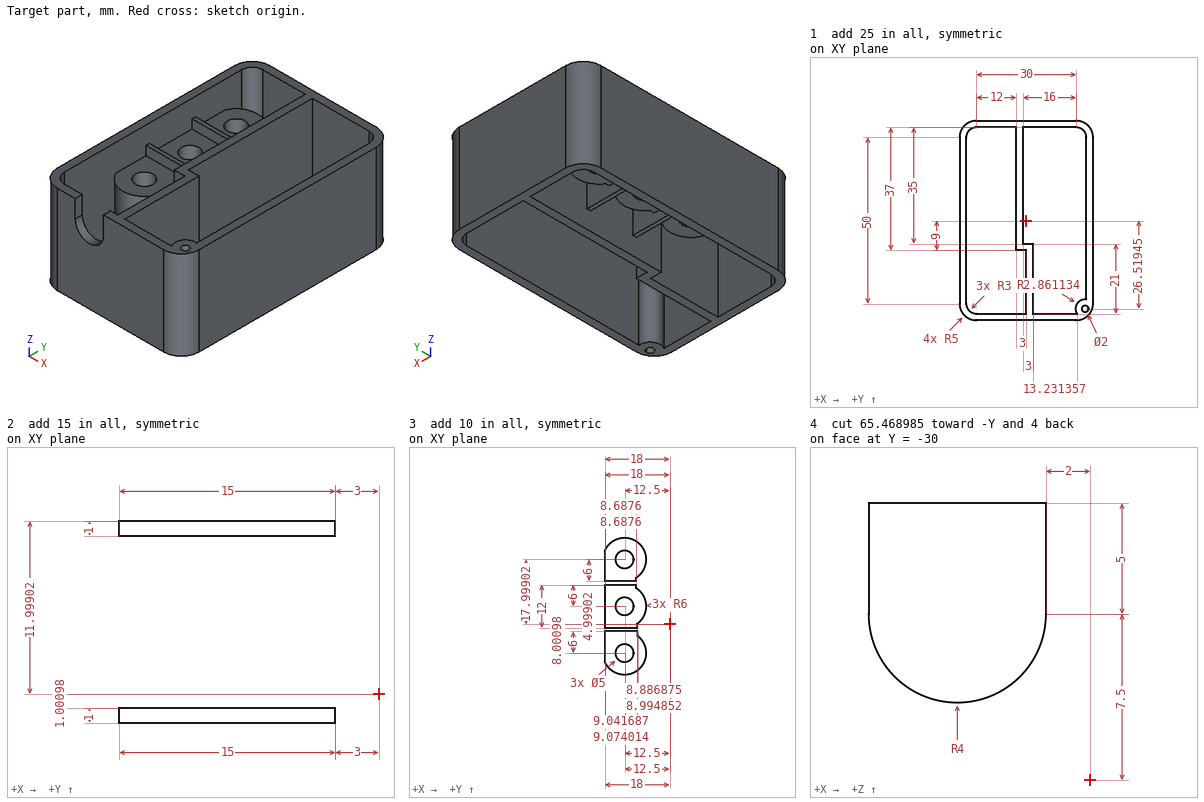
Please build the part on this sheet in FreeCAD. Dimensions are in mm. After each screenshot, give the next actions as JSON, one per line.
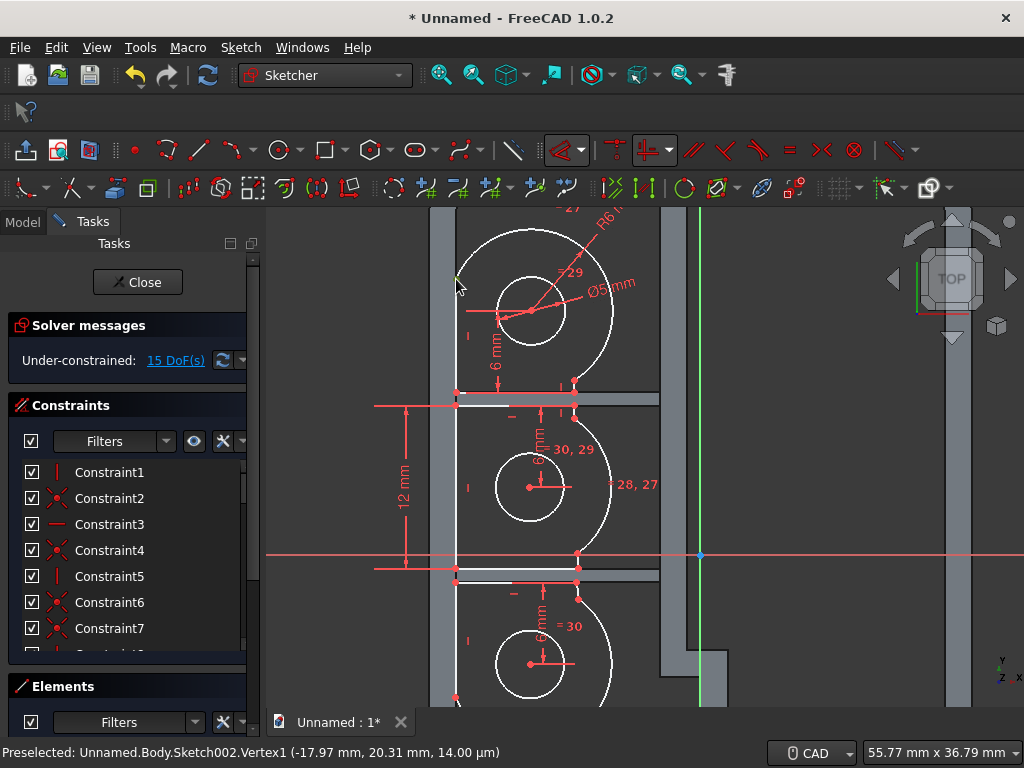
{"action": "key", "text": "l"}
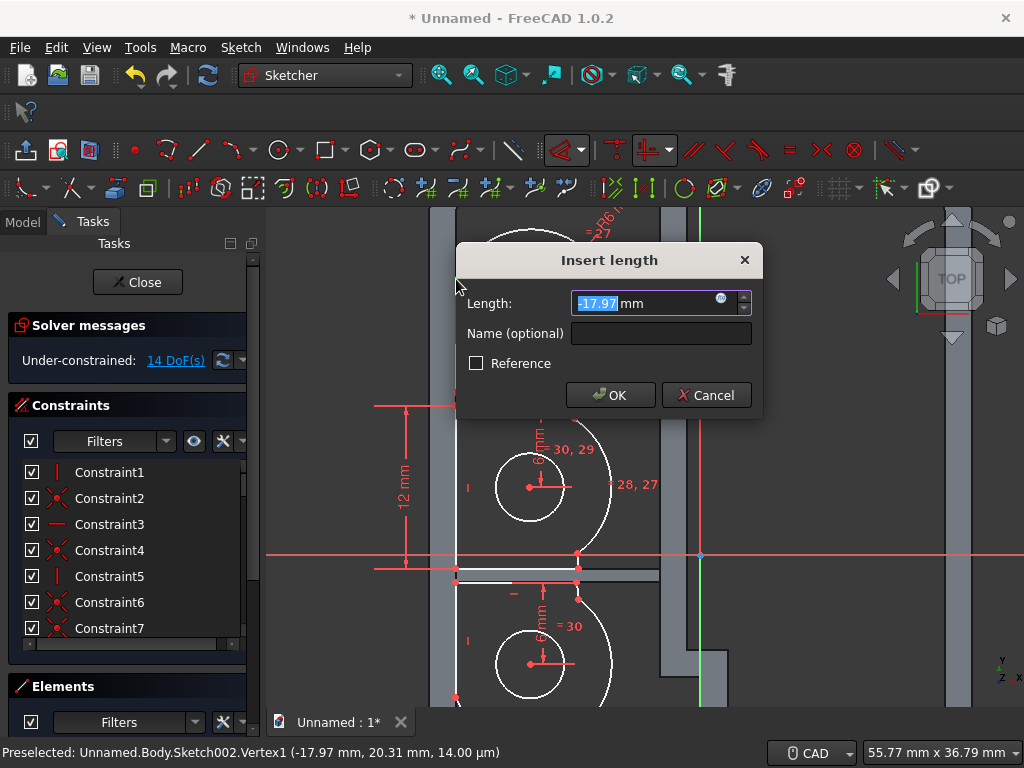
{"action": "type", "text": "-18"}
{"action": "key", "text": "Return"}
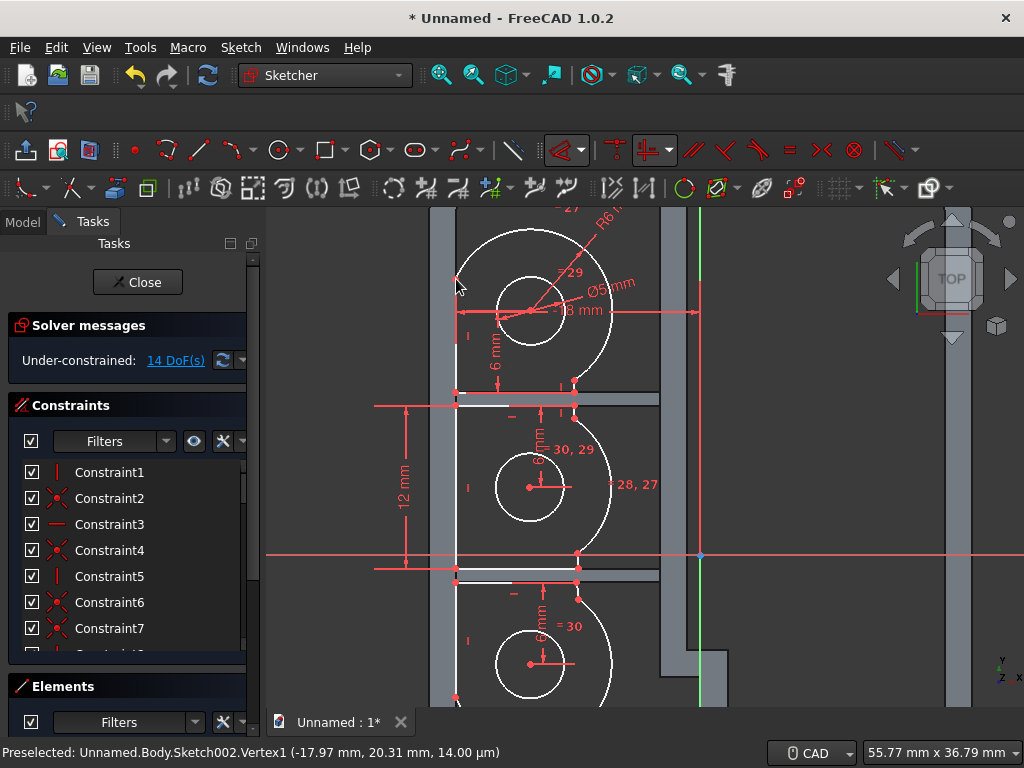
{"action": "left_click", "coordinate": [456, 406]}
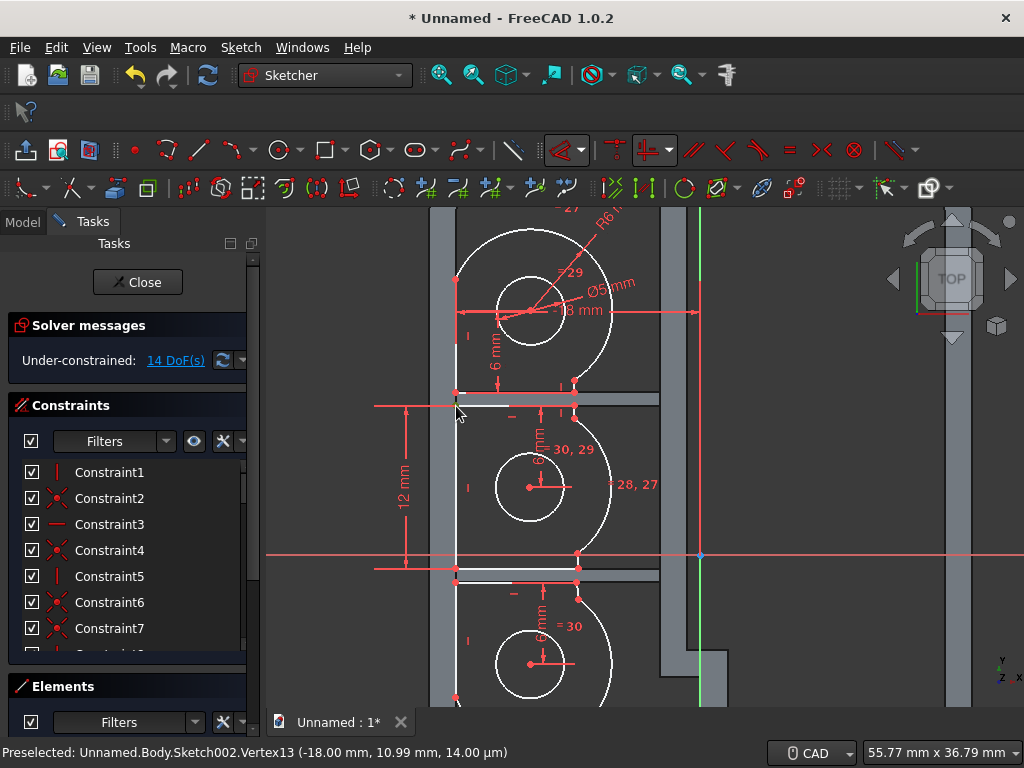
{"action": "left_click", "coordinate": [584, 150]}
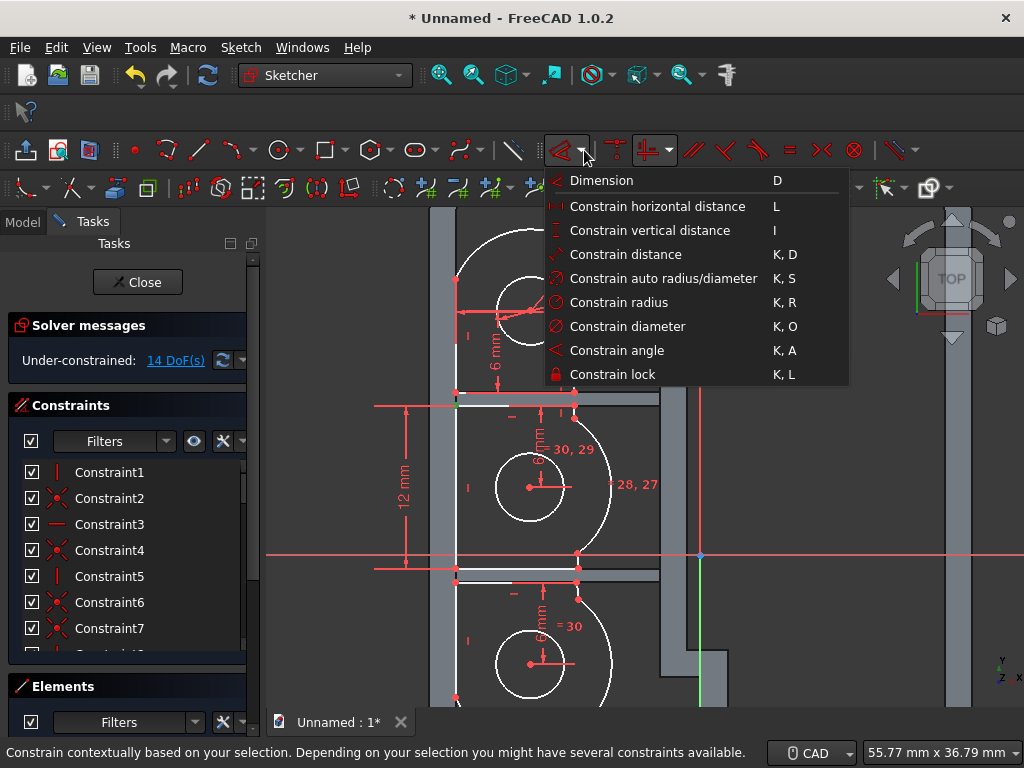
{"action": "left_click", "coordinate": [697, 206]}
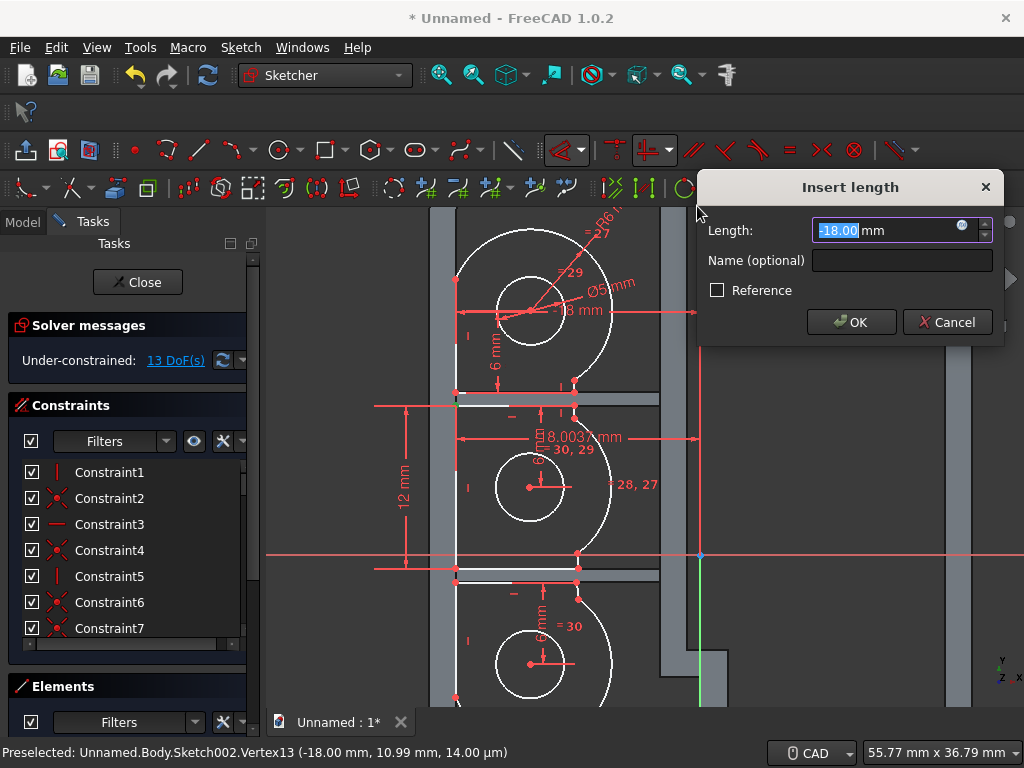
{"action": "type", "text": "-18"}
{"action": "key", "text": "Return"}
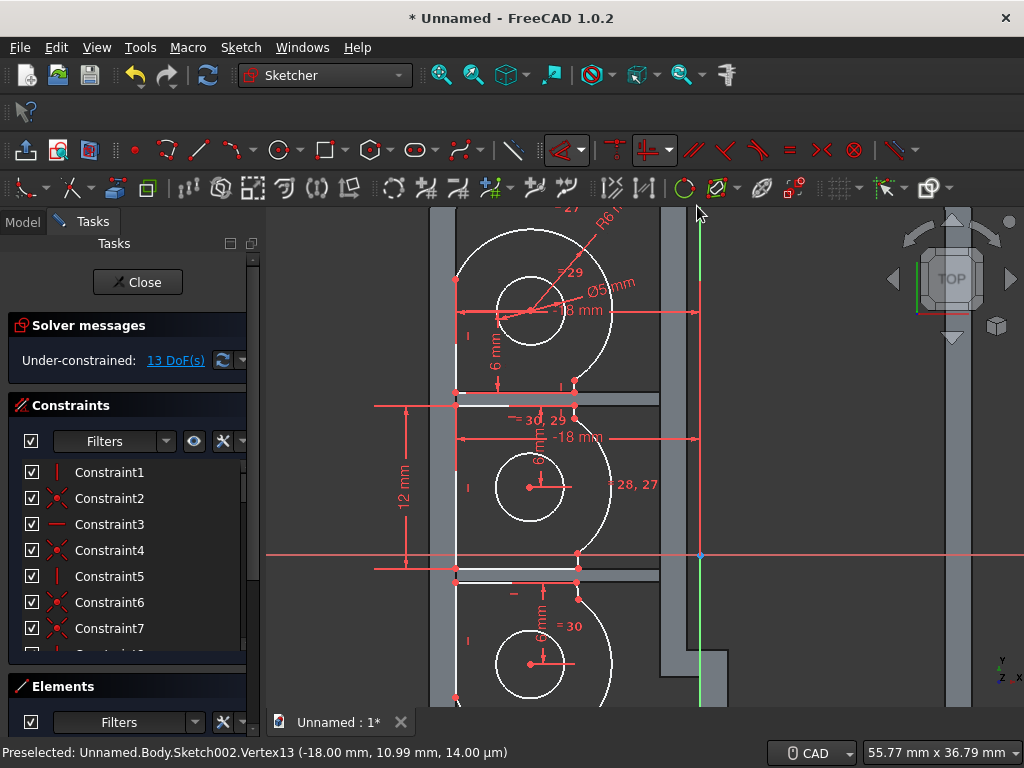
{"action": "left_click", "coordinate": [456, 583]}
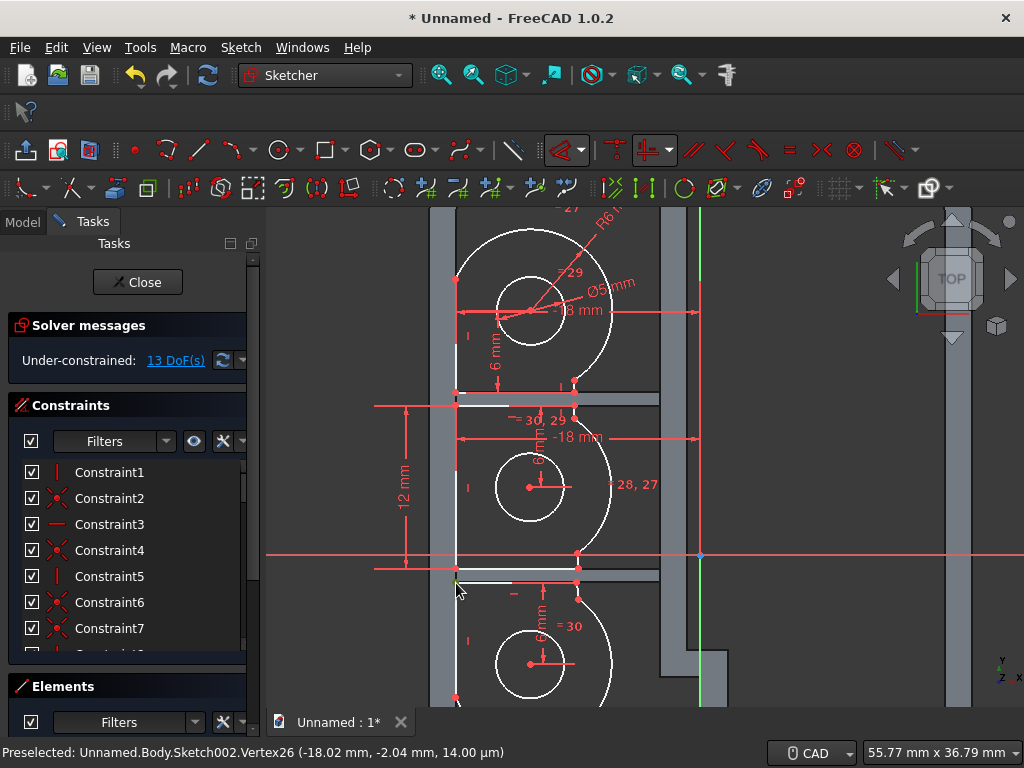
{"action": "key", "text": "l"}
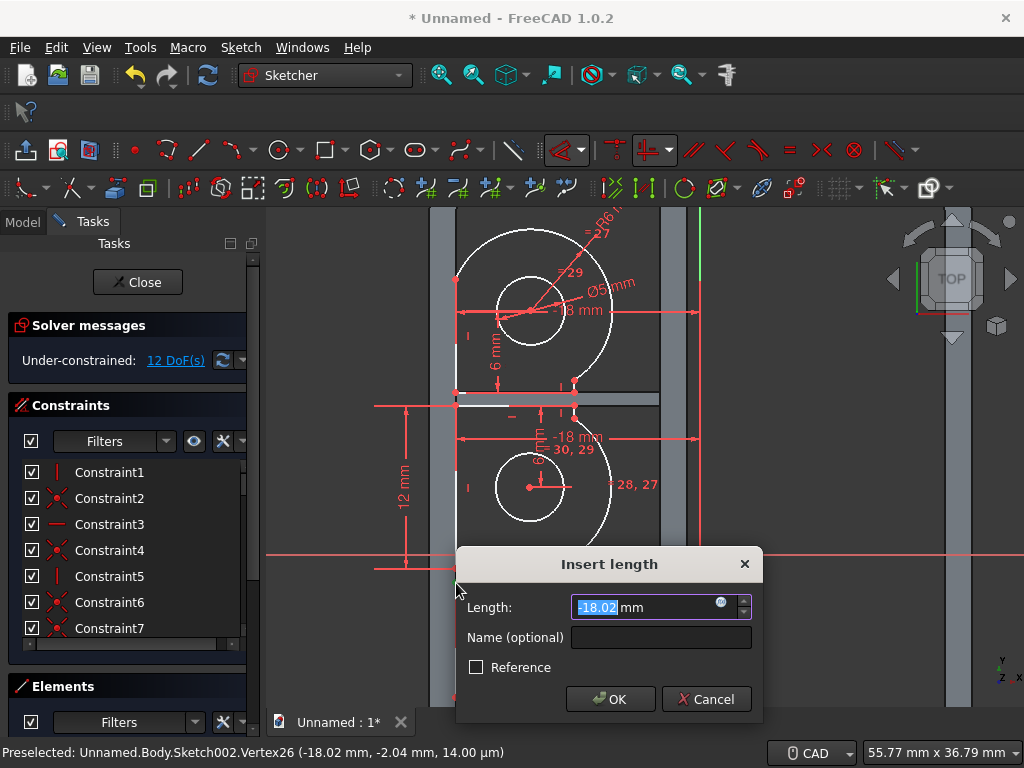
{"action": "type", "text": "-18"}
{"action": "key", "text": "Return"}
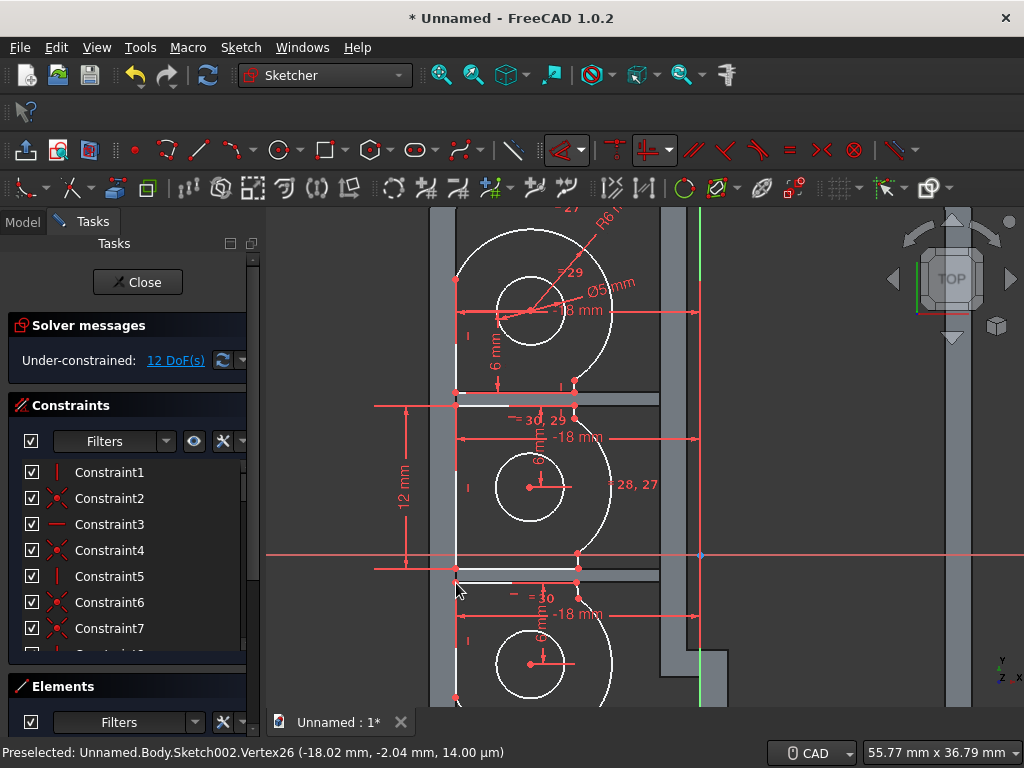
{"action": "left_click", "coordinate": [531, 311]}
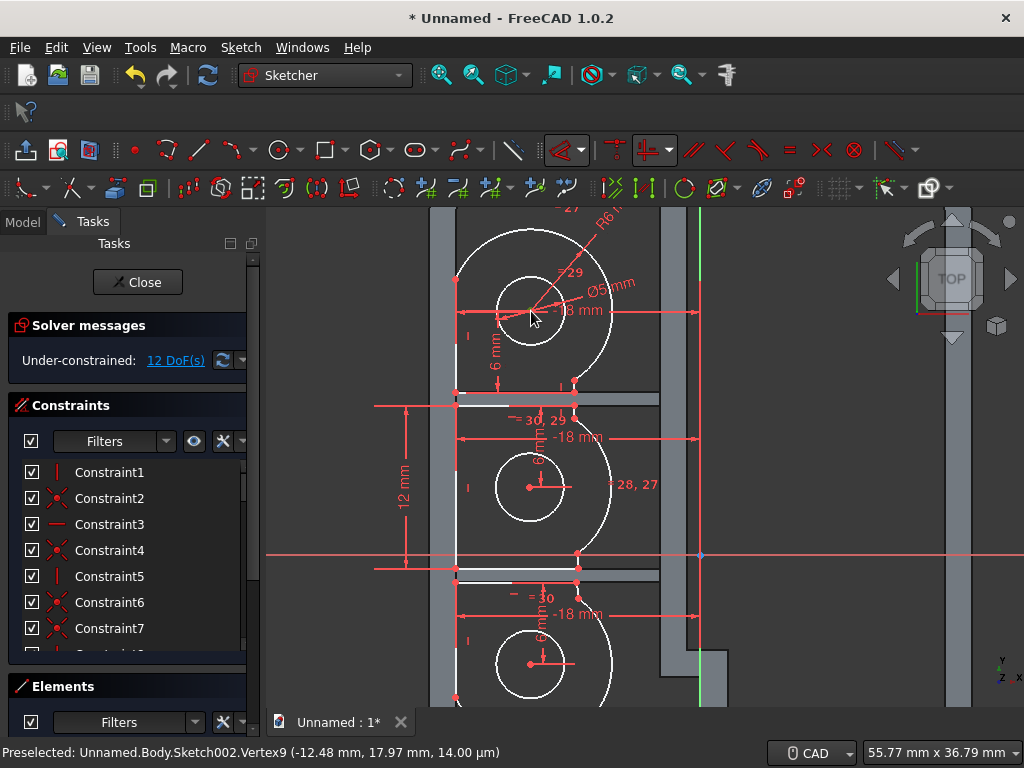
{"action": "left_click", "coordinate": [584, 150]}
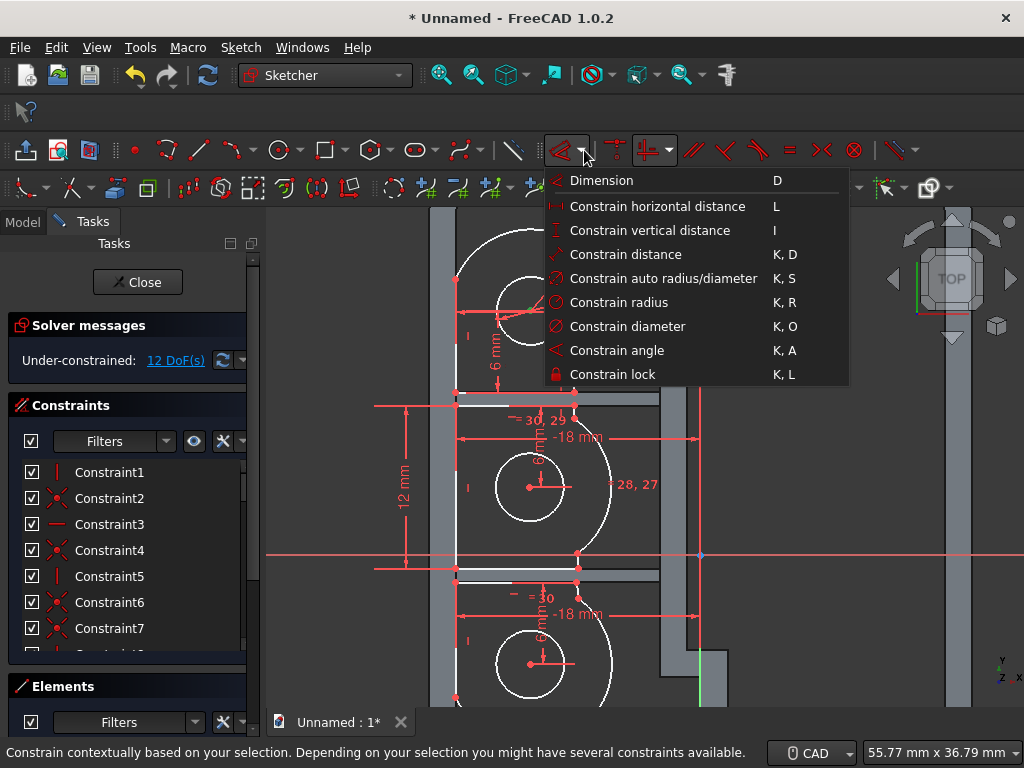
{"action": "left_click", "coordinate": [697, 206]}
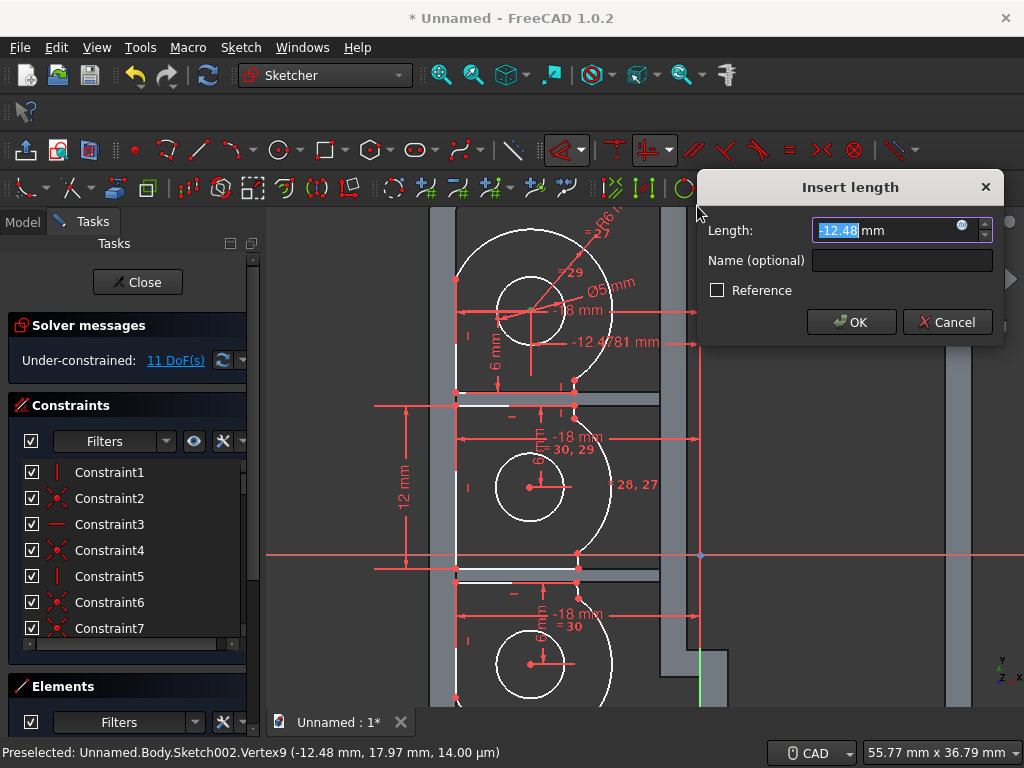
{"action": "type", "text": "-12.5"}
{"action": "key", "text": "Return"}